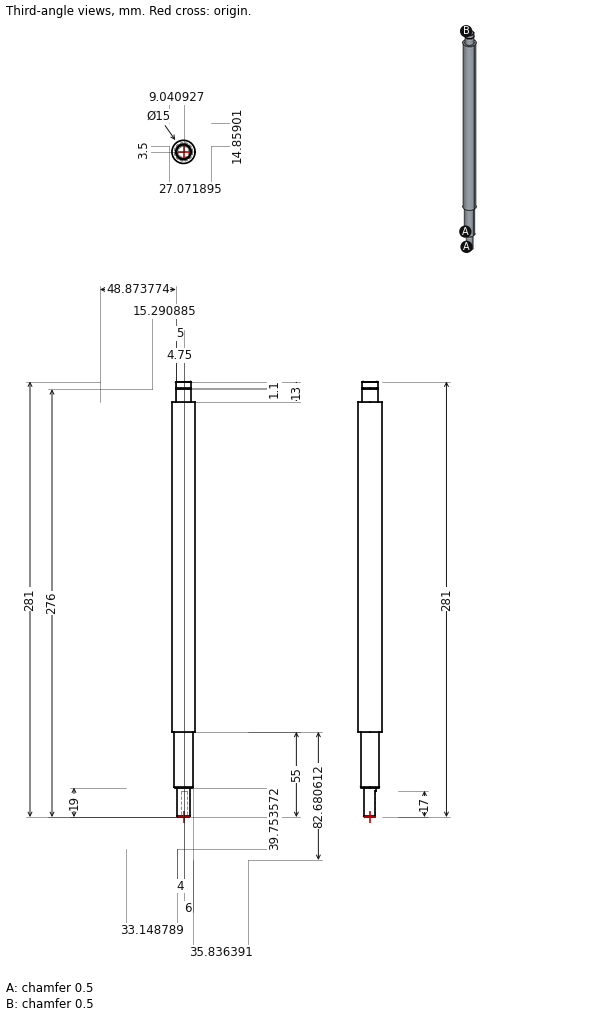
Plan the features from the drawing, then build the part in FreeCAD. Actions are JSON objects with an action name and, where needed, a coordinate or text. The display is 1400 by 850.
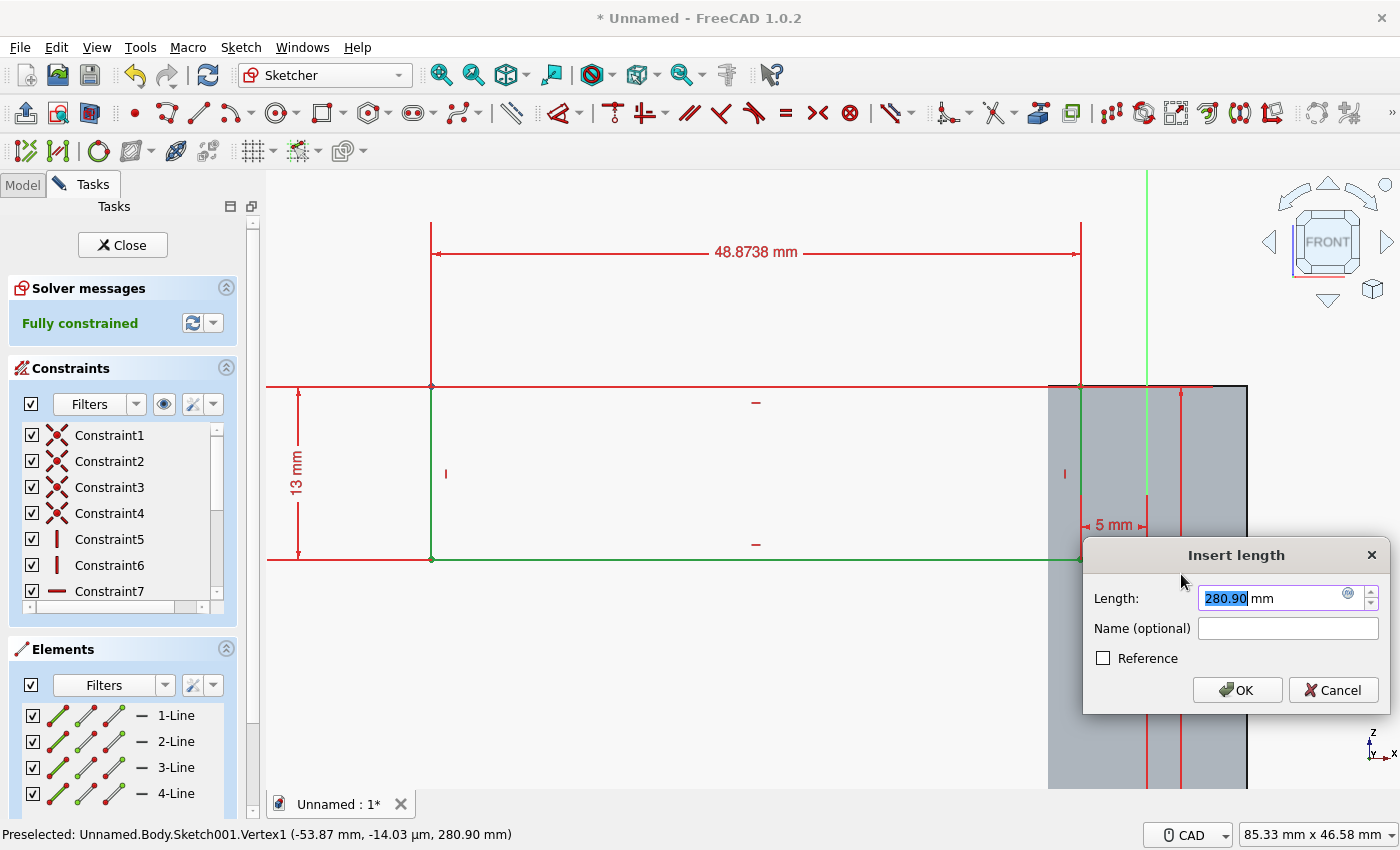
{"action": "type", "text": "281"}
{"action": "key", "text": "Return"}
{"action": "key", "text": "Escape"}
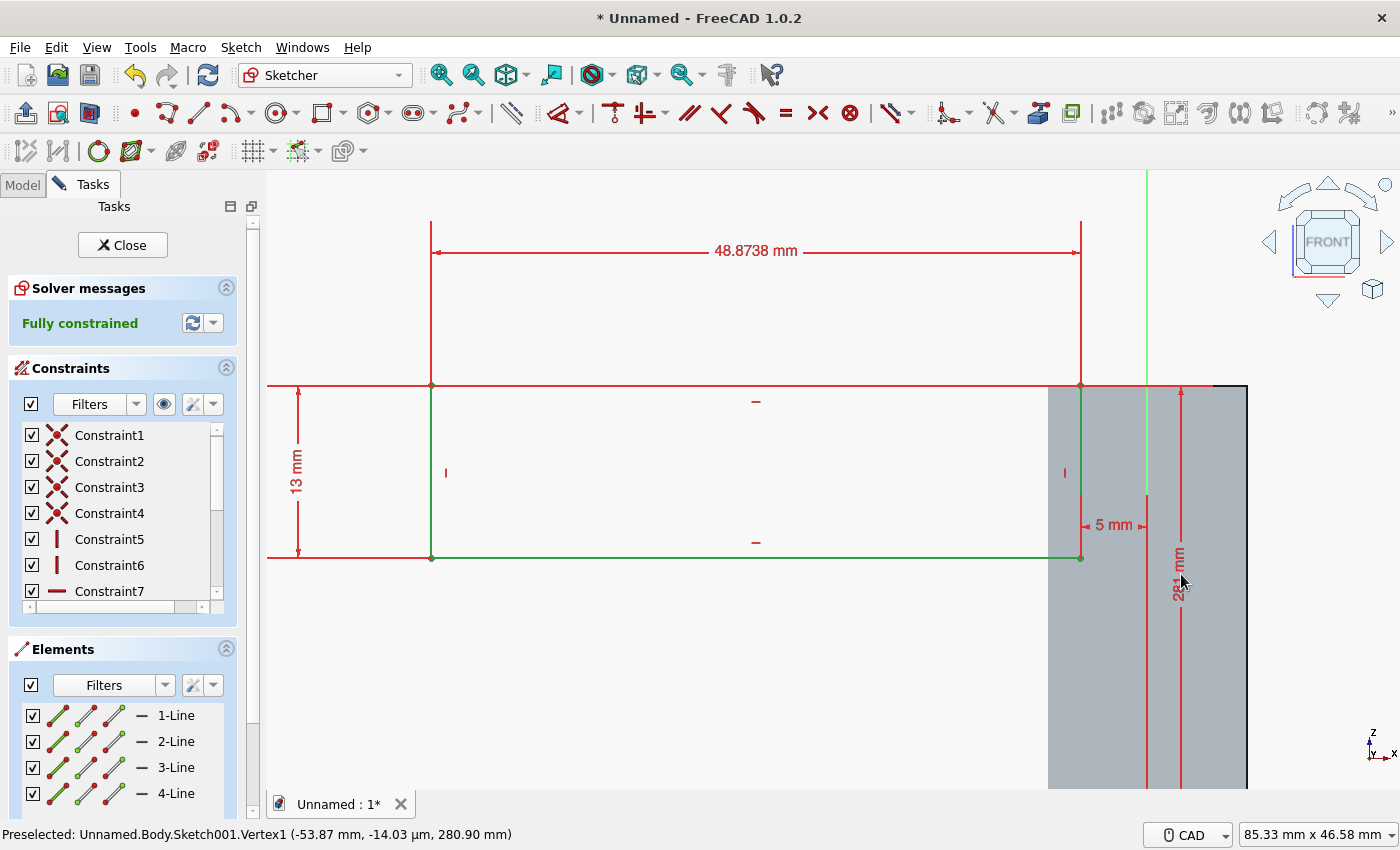
{"action": "left_click", "coordinate": [123, 245]}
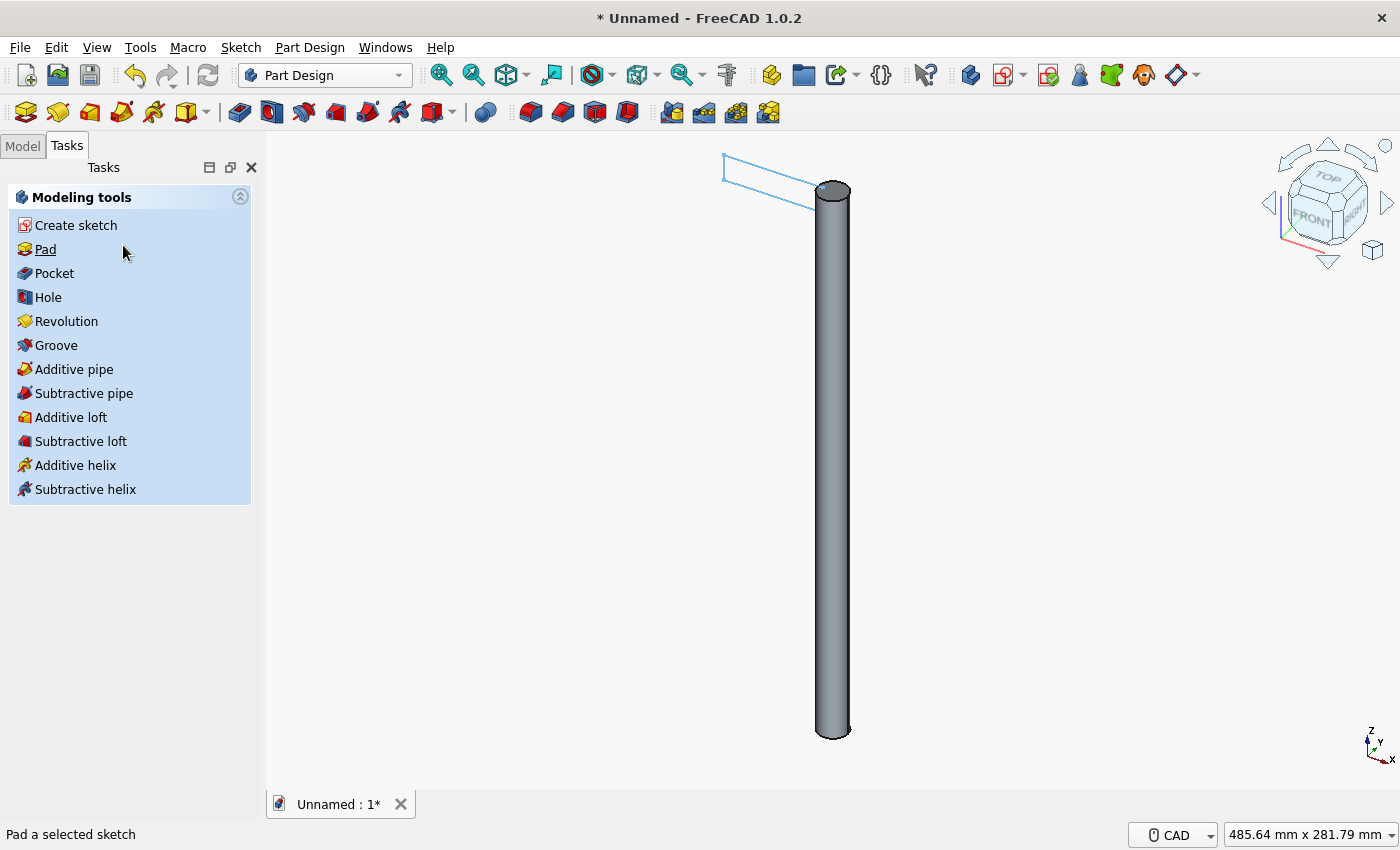
{"action": "left_click", "coordinate": [304, 112]}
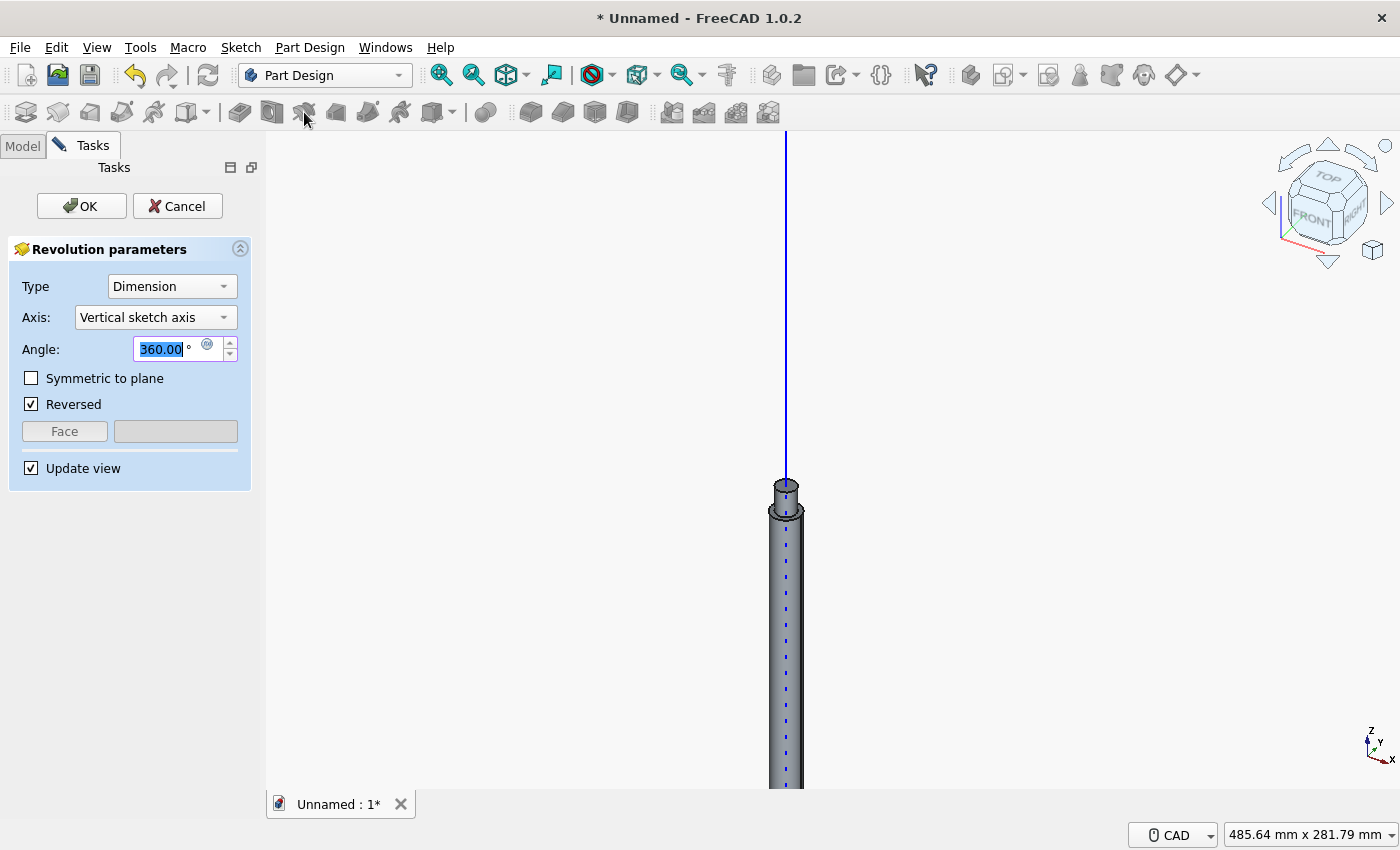
{"action": "left_click", "coordinate": [82, 206]}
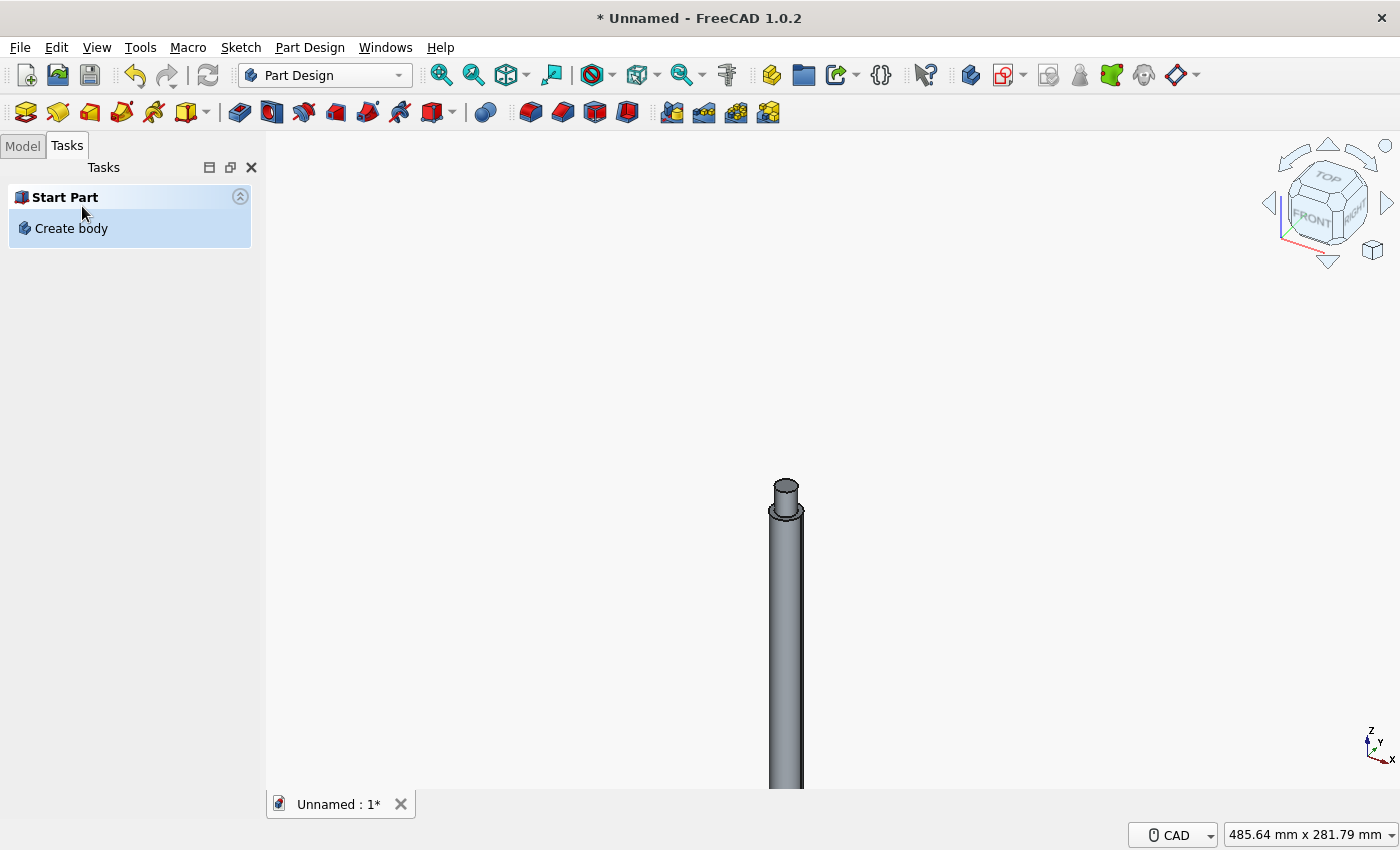
{"action": "left_click", "coordinate": [442, 76]}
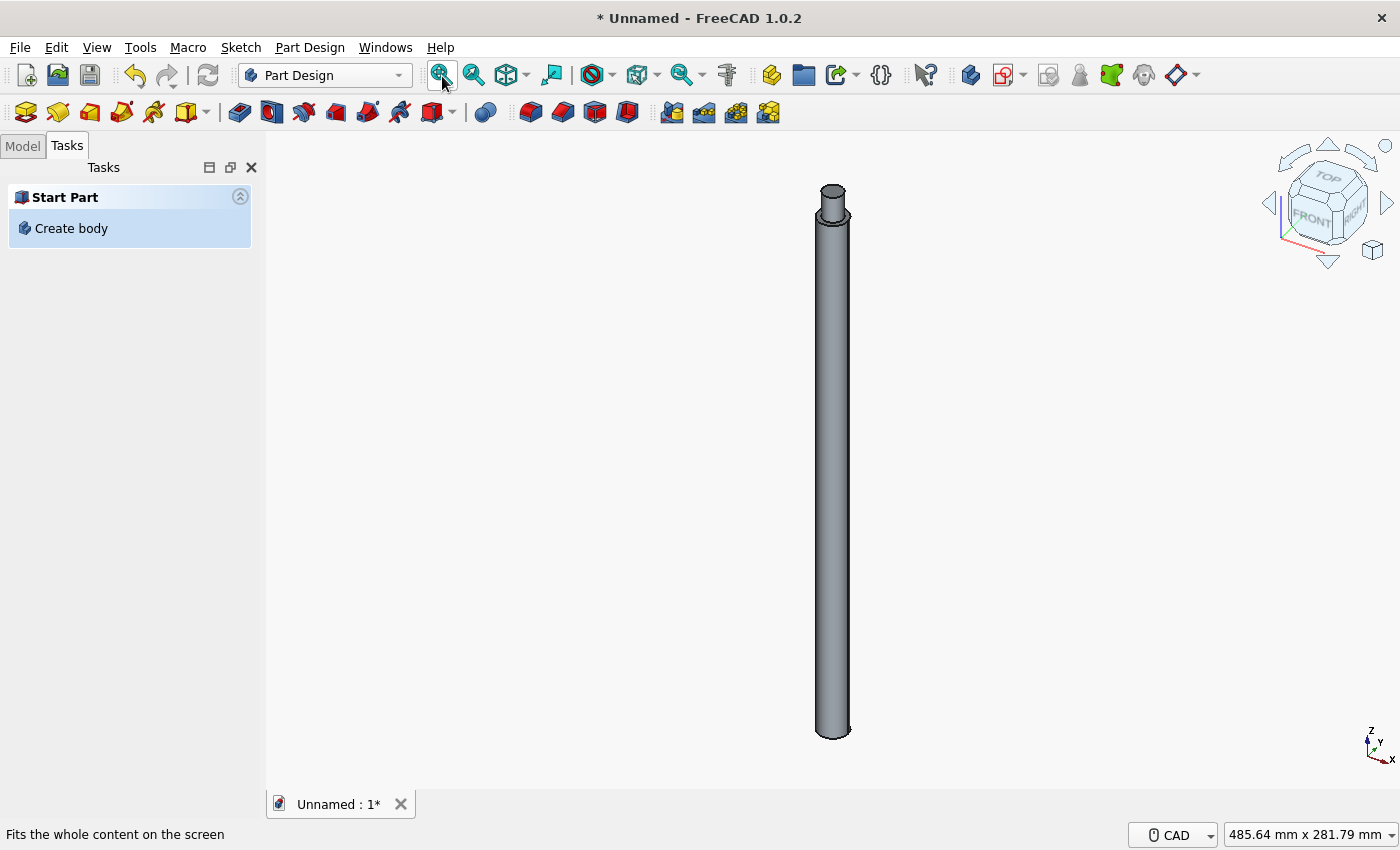
{"action": "left_click", "coordinate": [1004, 76]}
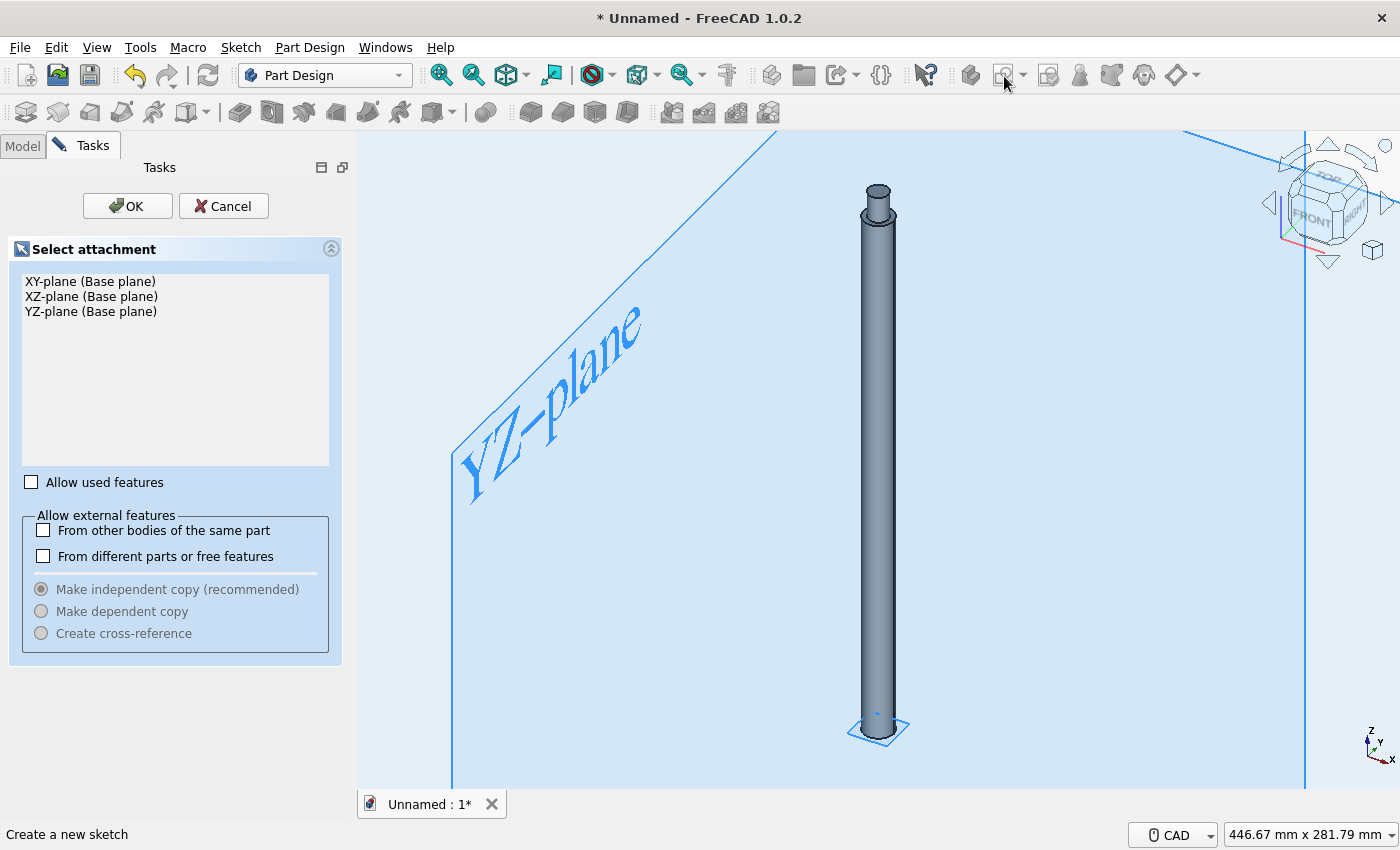
{"action": "left_click", "coordinate": [82, 296]}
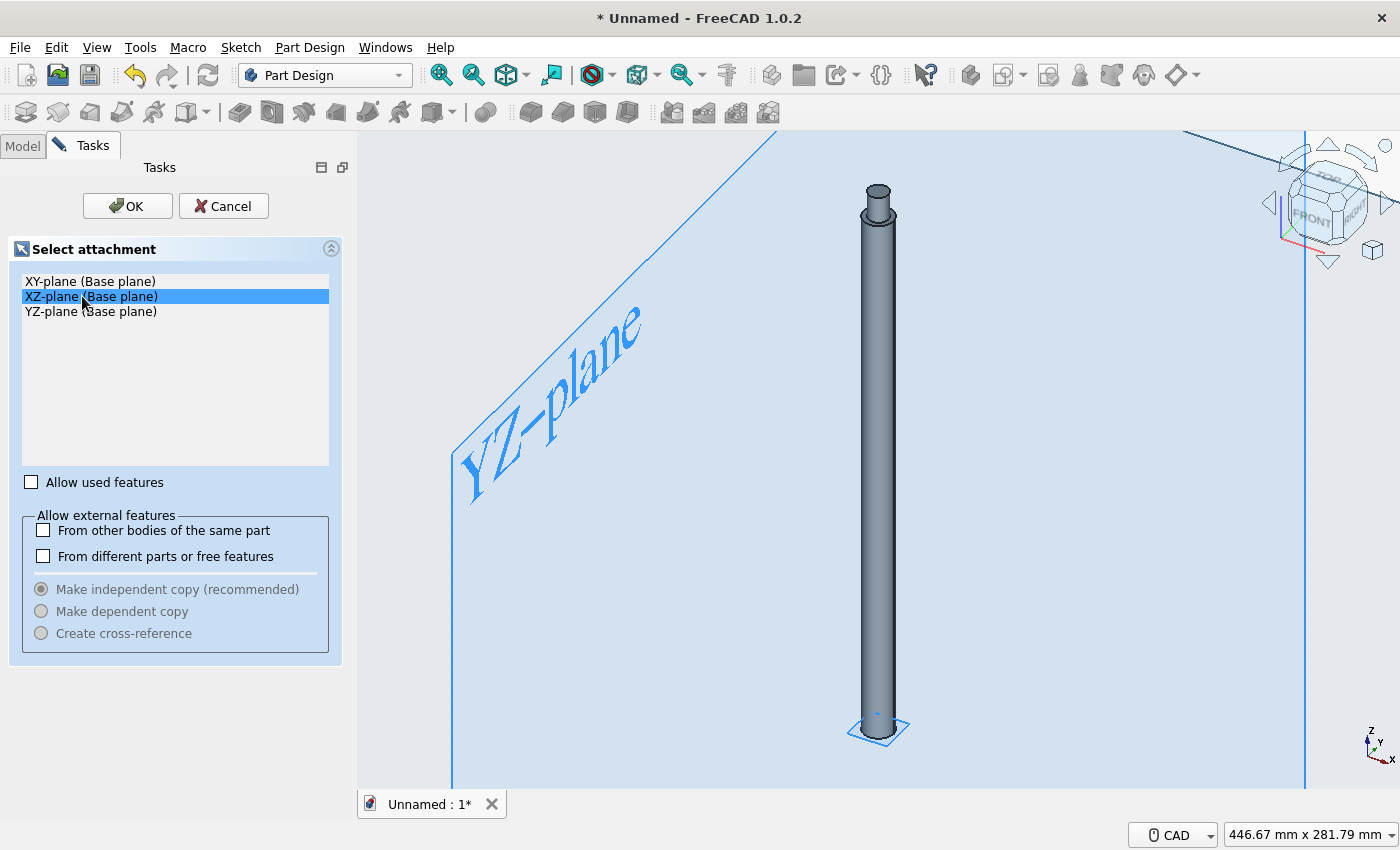
{"action": "left_click", "coordinate": [128, 206]}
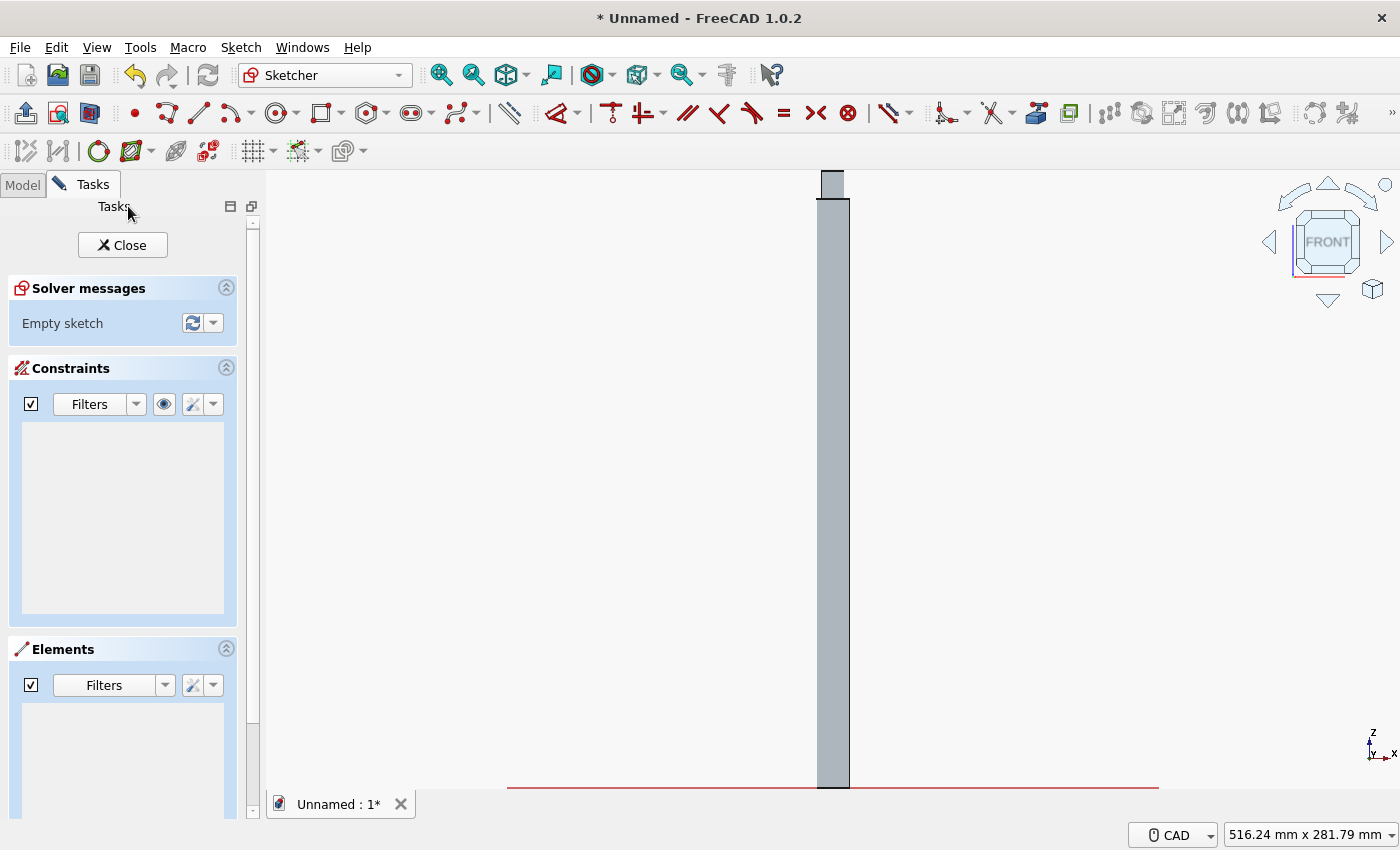
{"action": "left_click", "coordinate": [90, 114]}